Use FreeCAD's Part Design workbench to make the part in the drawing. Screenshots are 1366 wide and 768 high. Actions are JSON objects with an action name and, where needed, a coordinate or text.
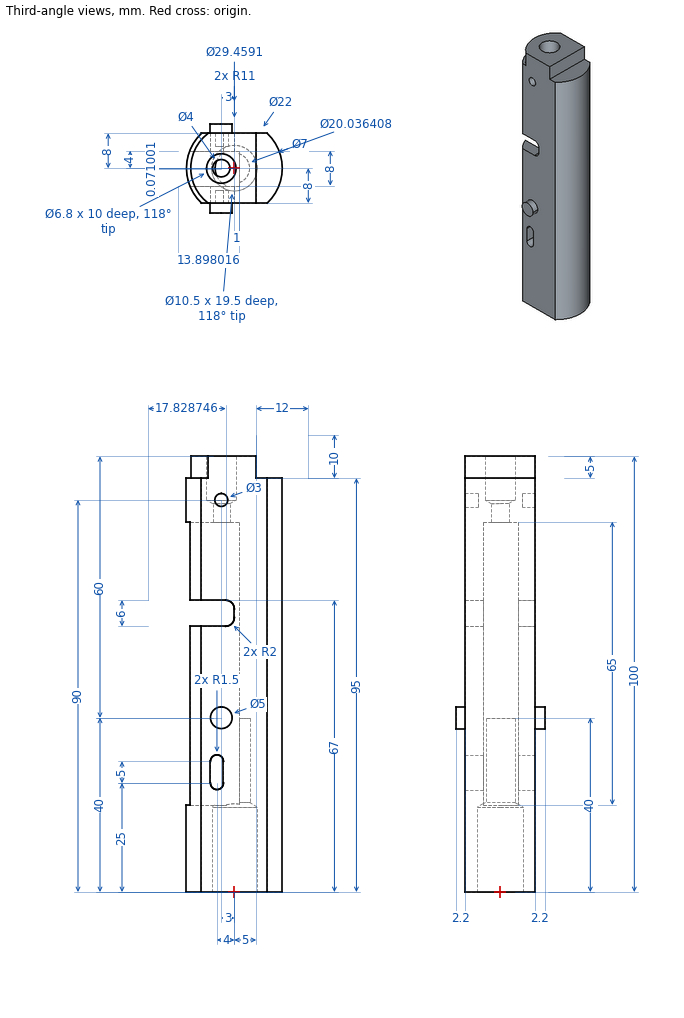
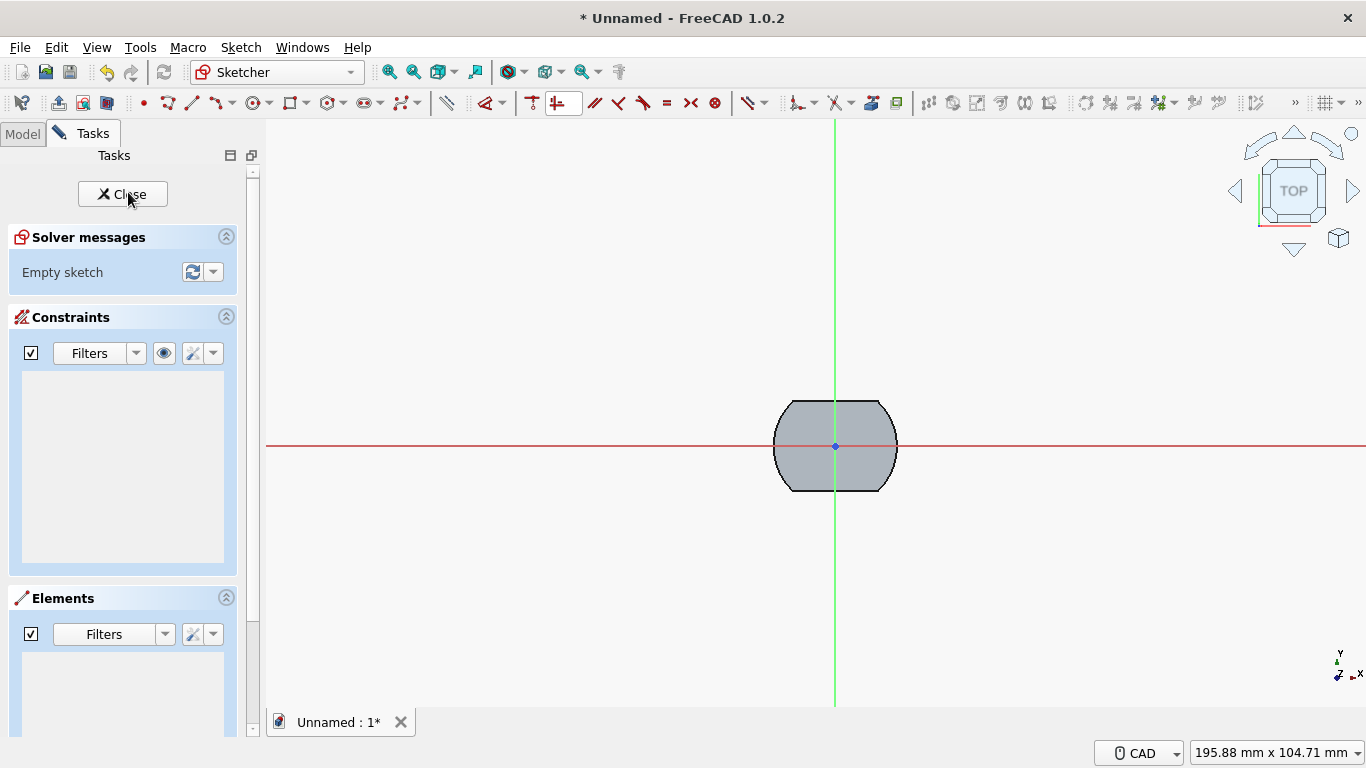
{"action": "scroll", "coordinate": [853, 453], "scroll_direction": "up", "scroll_amount": 9}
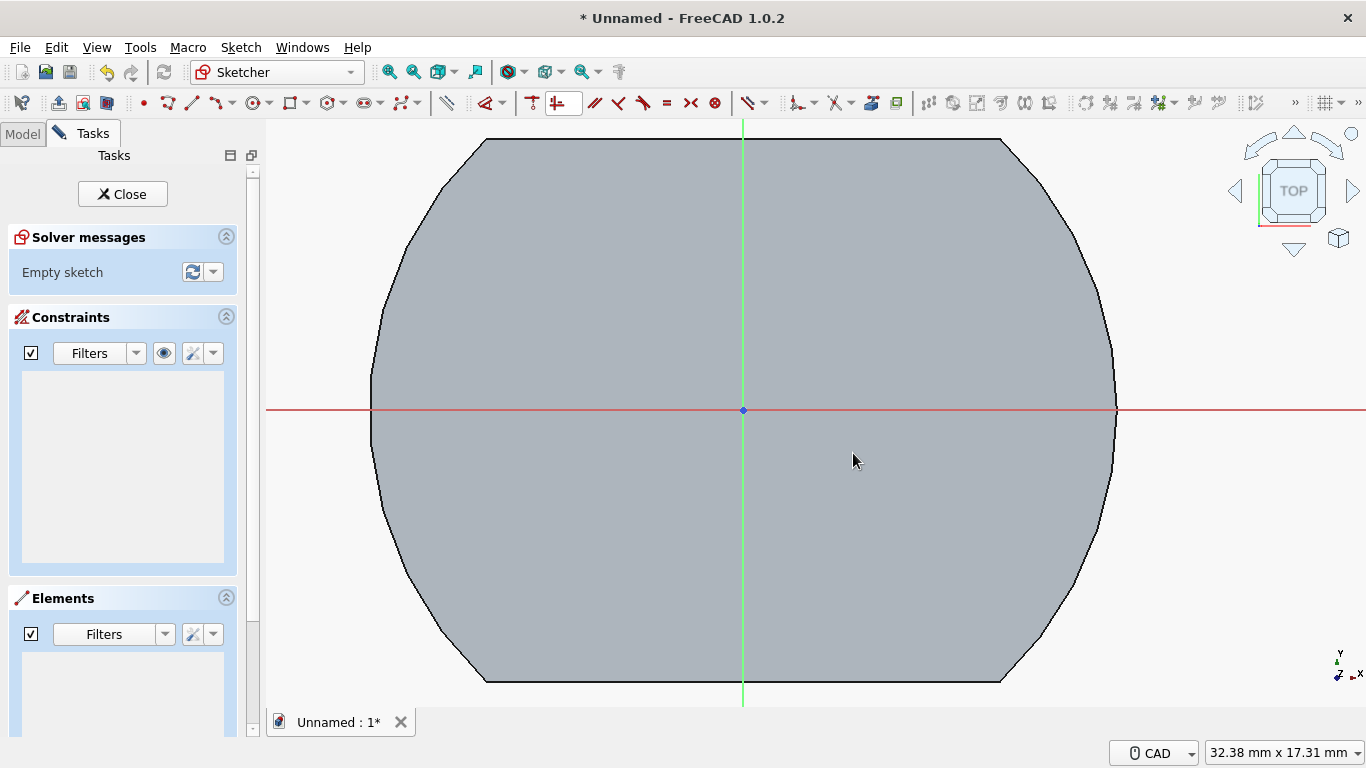
{"action": "left_click", "coordinate": [254, 104]}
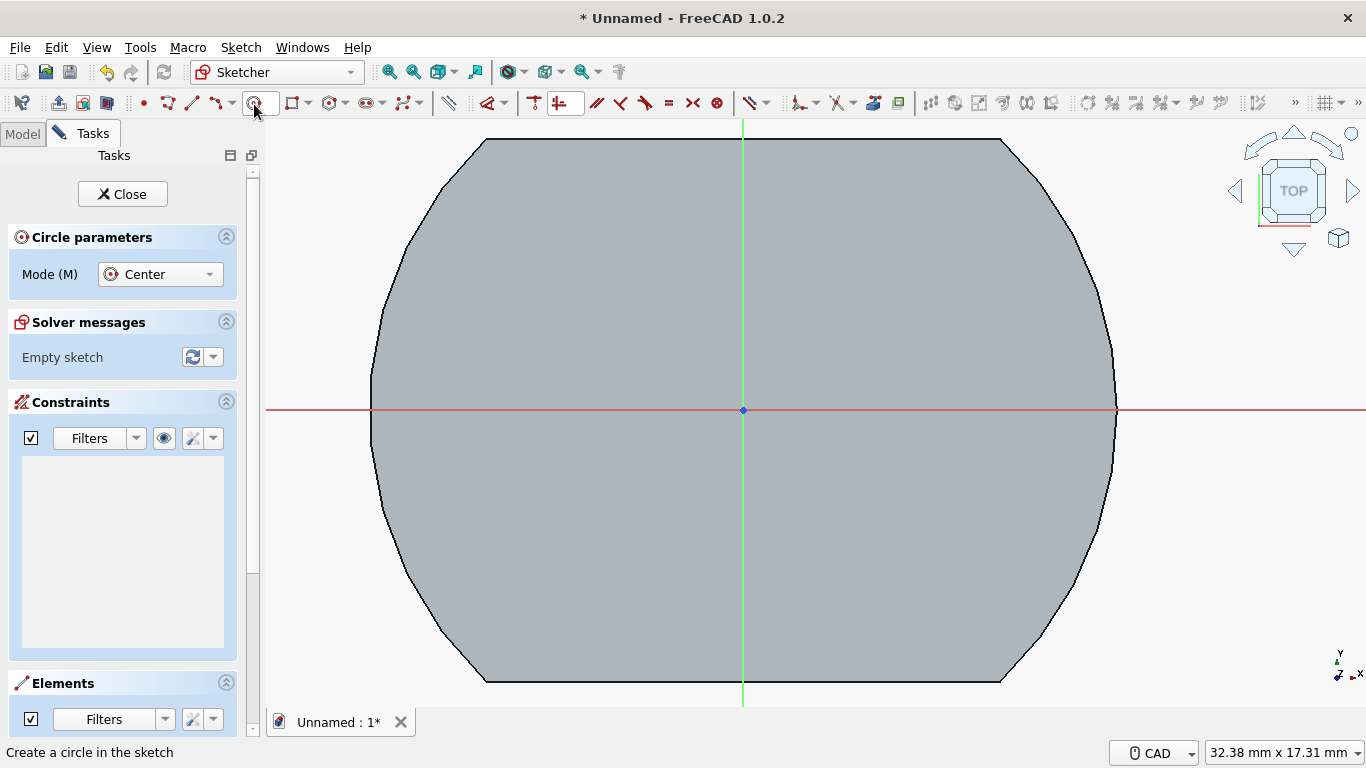
{"action": "left_click", "coordinate": [743, 410]}
{"action": "mouse_move", "coordinate": [869, 284]}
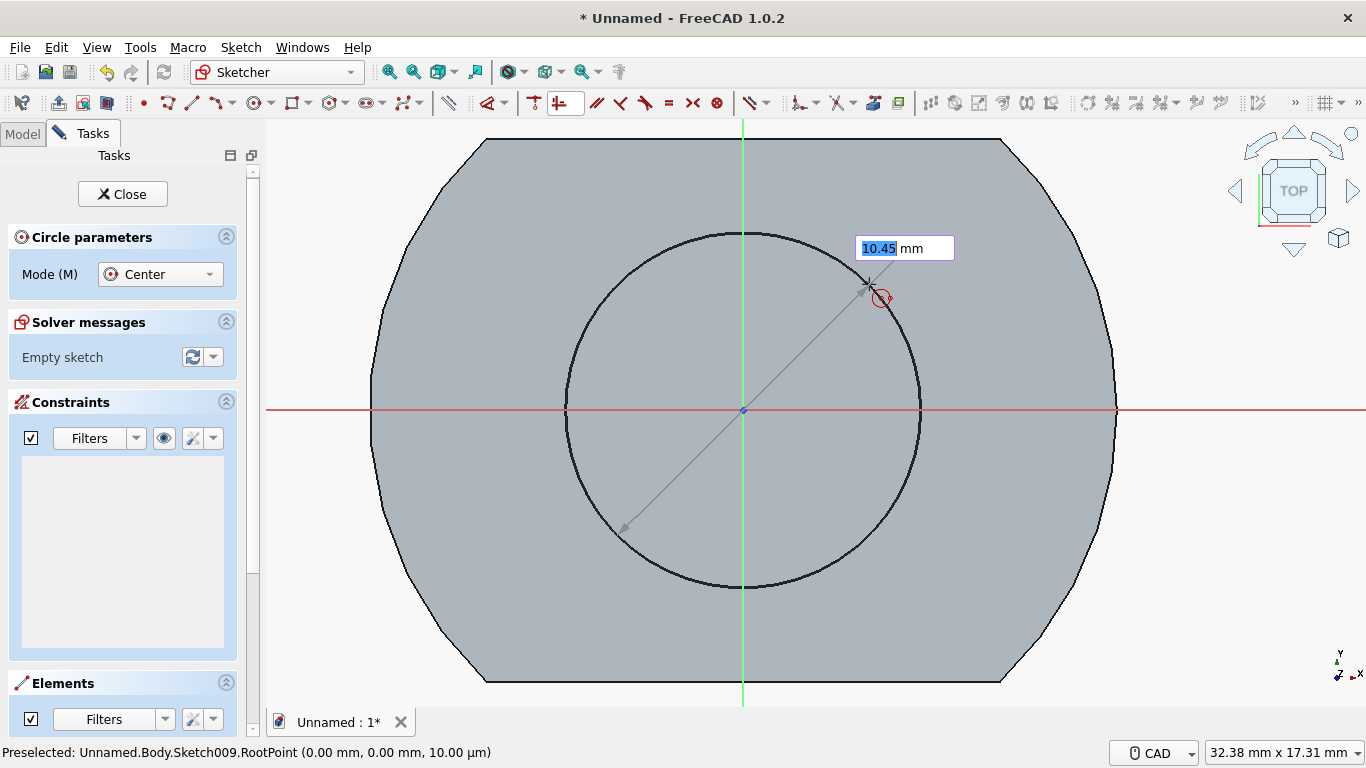
{"action": "type", "text": "10.5"}
{"action": "key", "text": "Return"}
{"action": "key", "text": "Escape"}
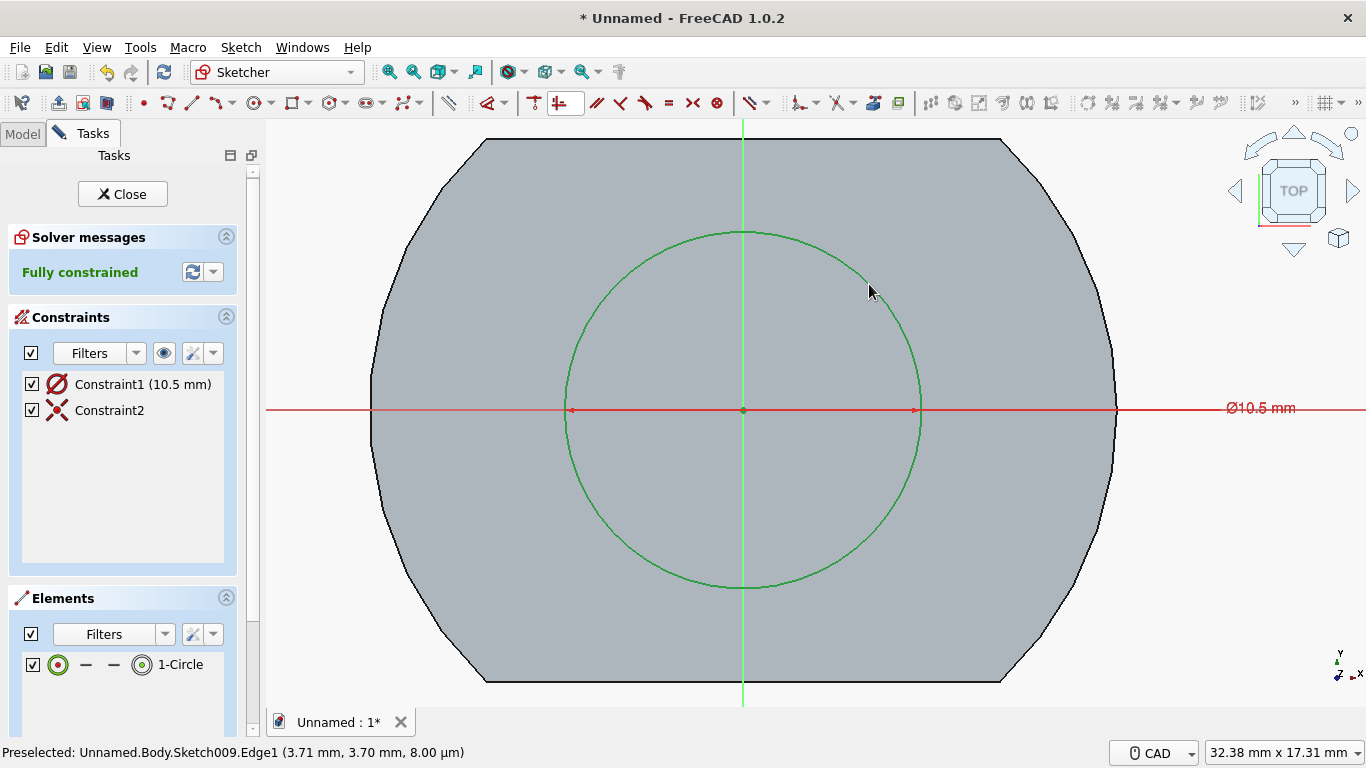
{"action": "left_click", "coordinate": [123, 194]}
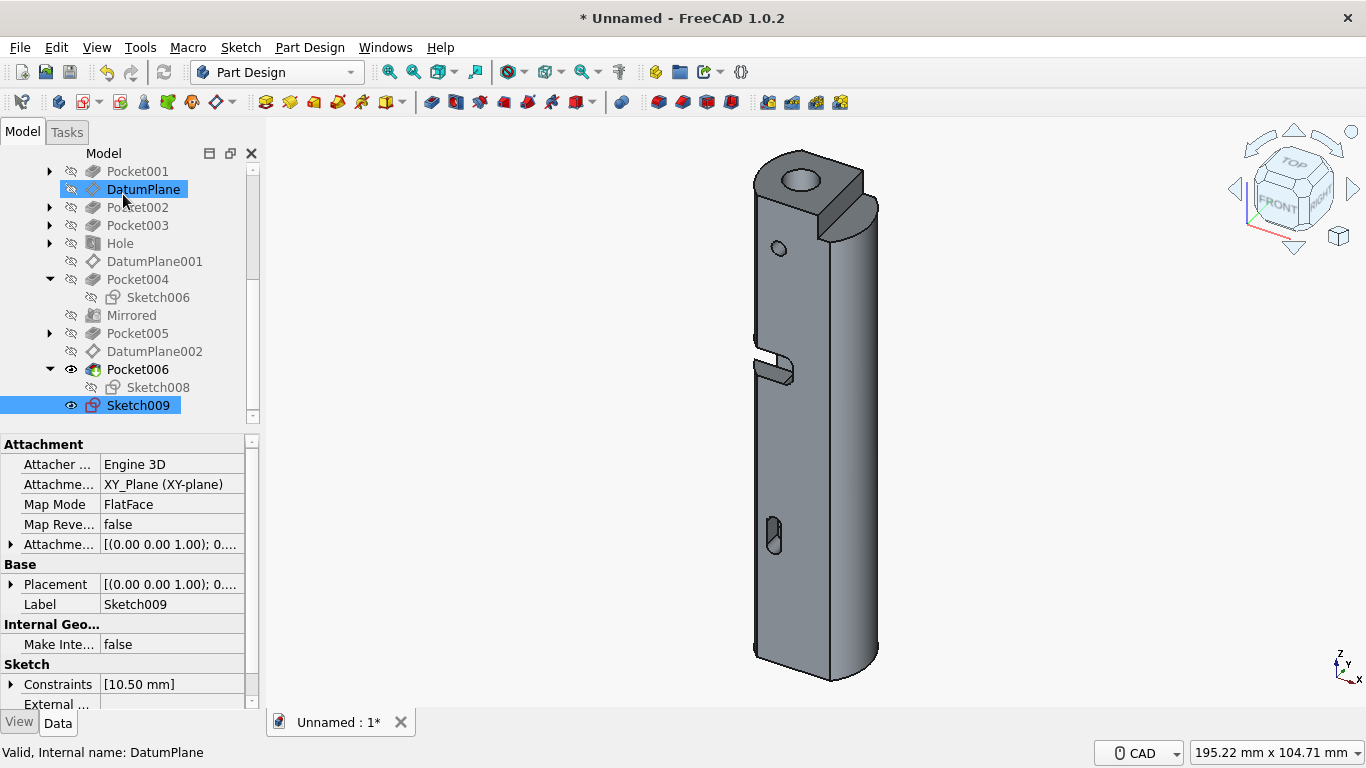
{"action": "left_click", "coordinate": [456, 102]}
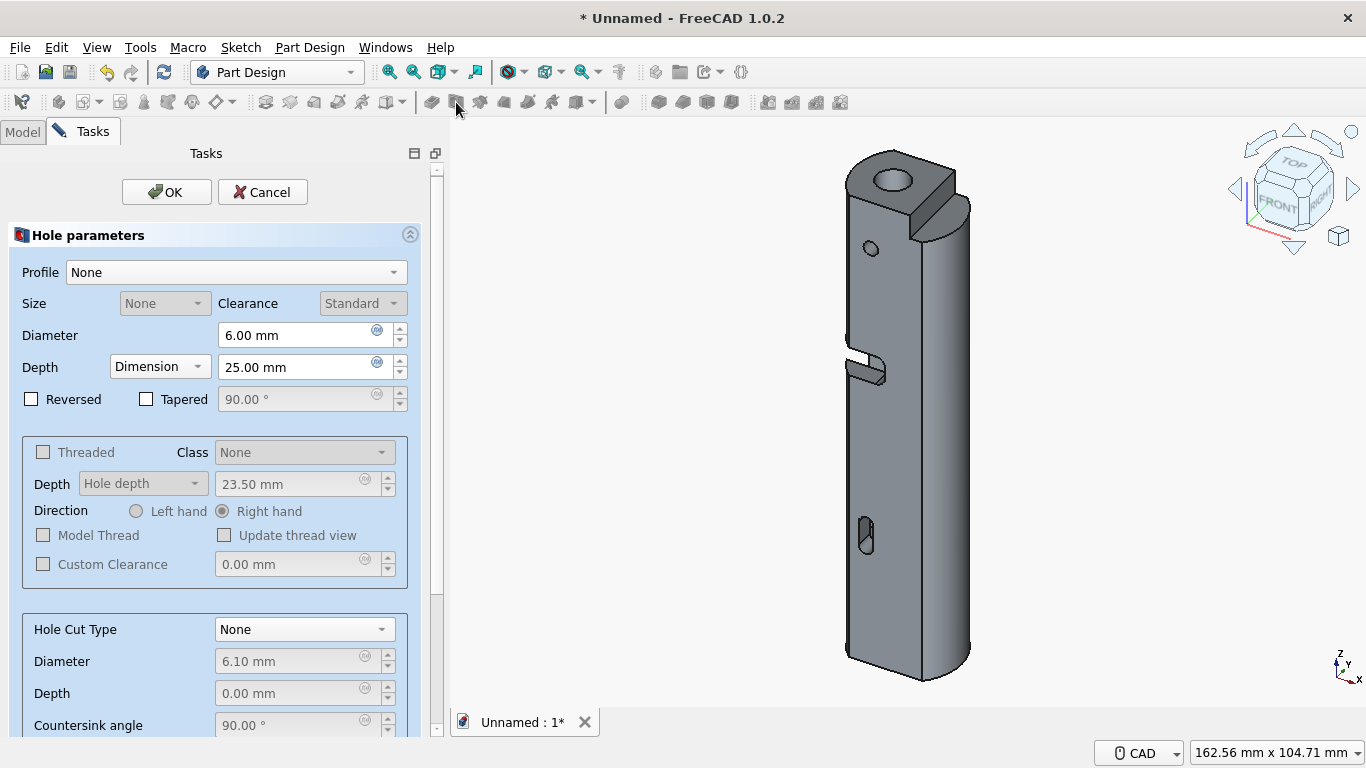
{"action": "triple_click", "coordinate": [305, 335]}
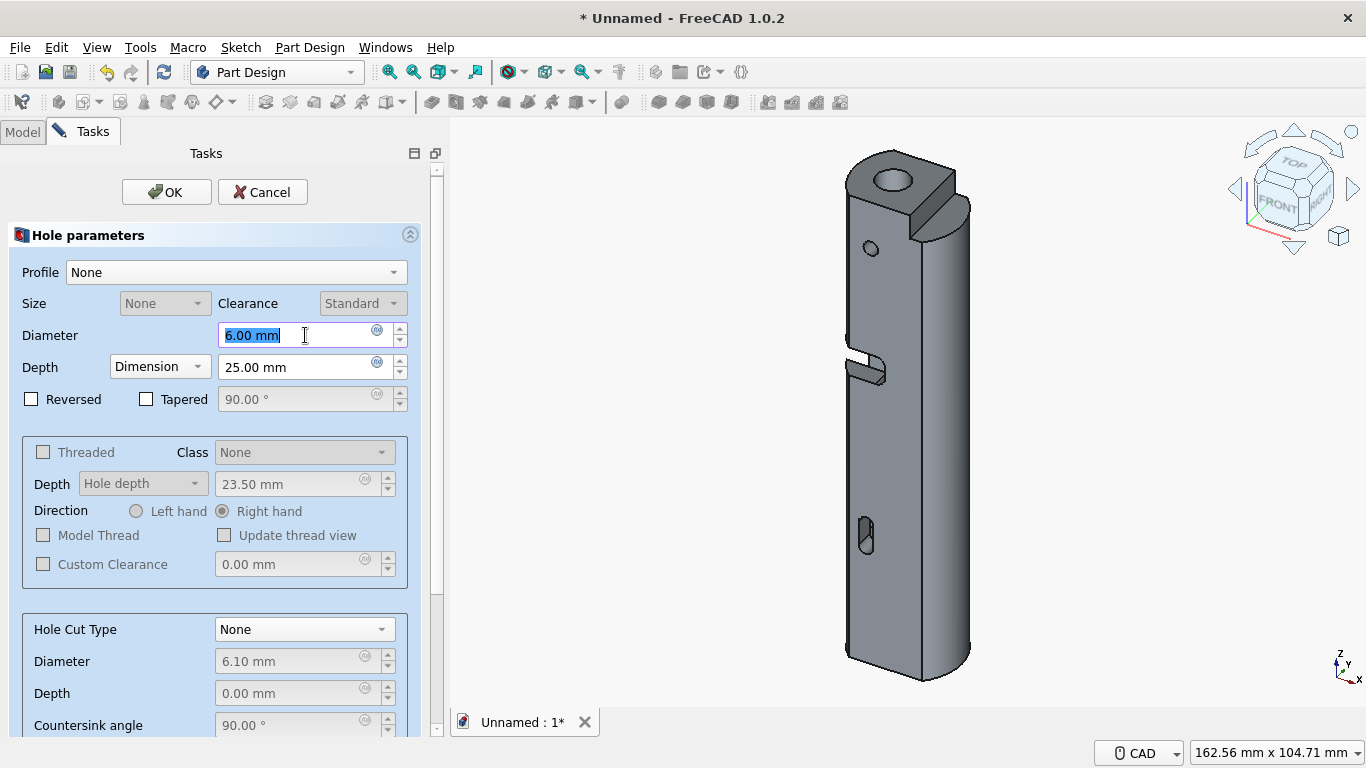
{"action": "type", "text": "10.5"}
{"action": "key", "text": "Tab"}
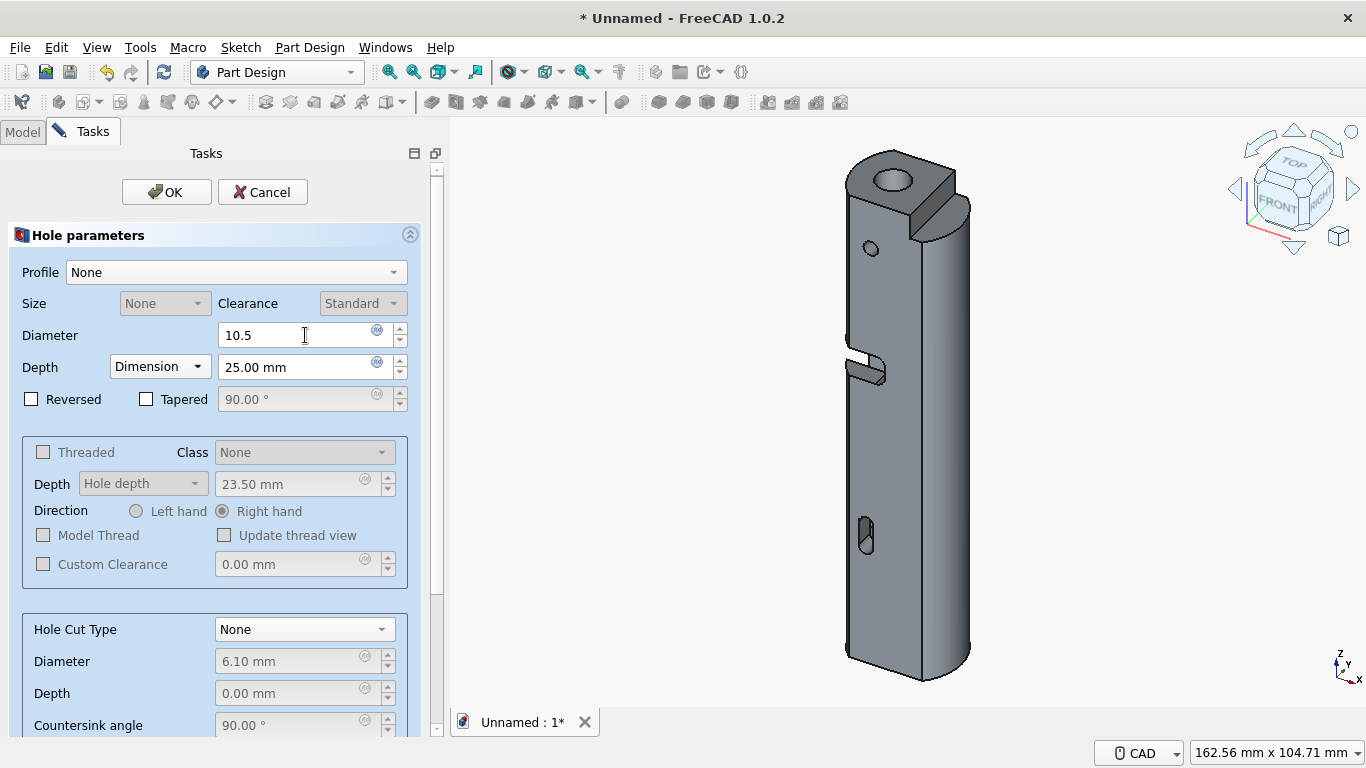
{"action": "triple_click", "coordinate": [305, 367]}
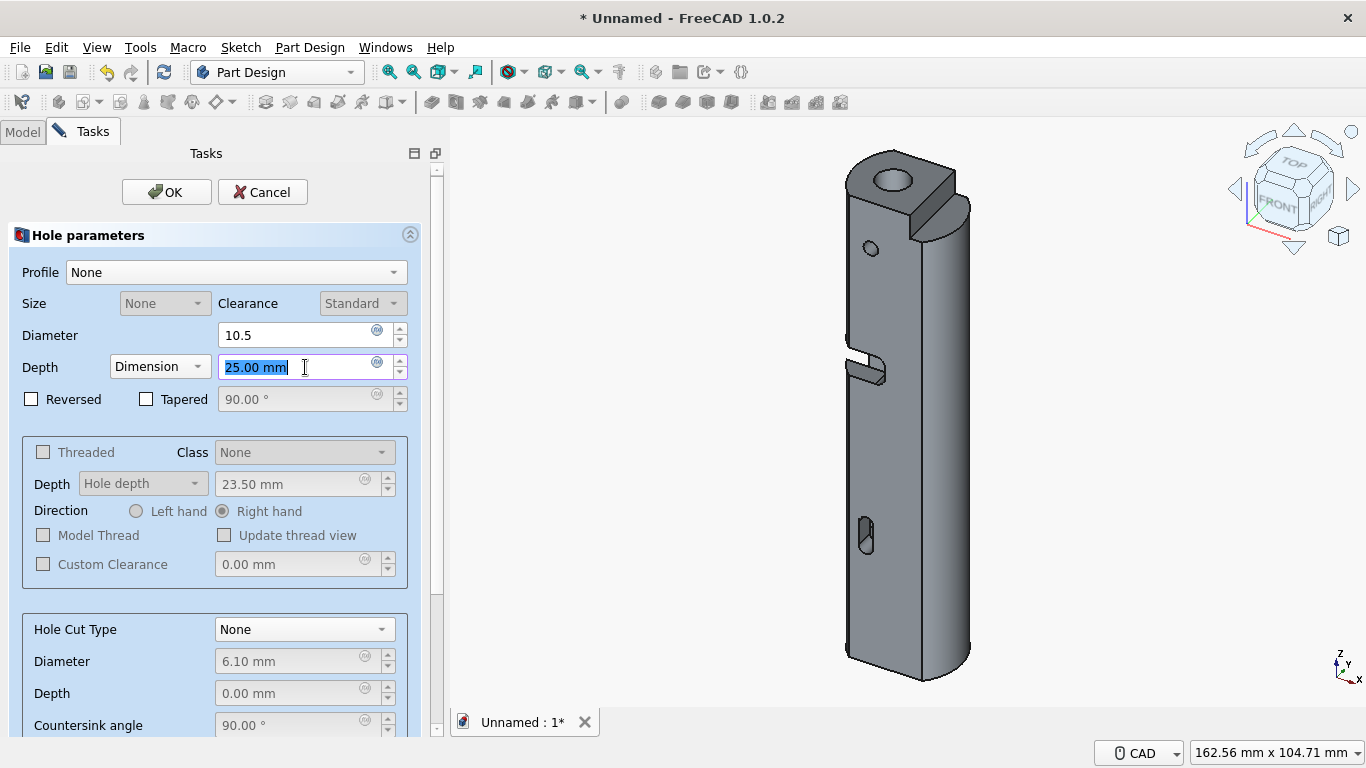
{"action": "type", "text": "19.5"}
{"action": "key", "text": "Tab"}